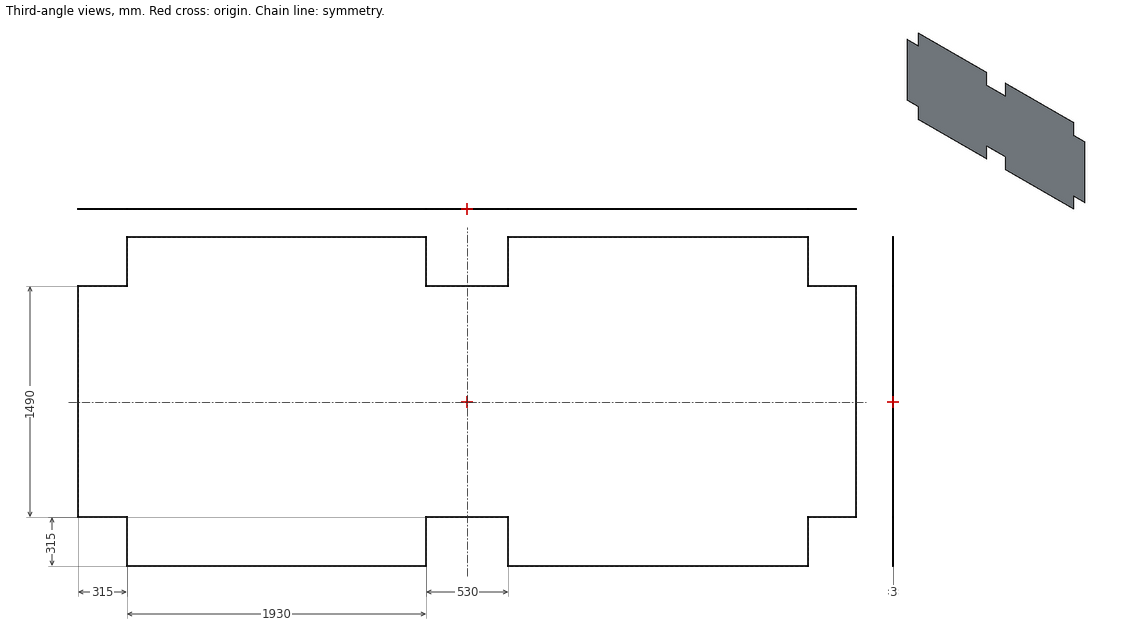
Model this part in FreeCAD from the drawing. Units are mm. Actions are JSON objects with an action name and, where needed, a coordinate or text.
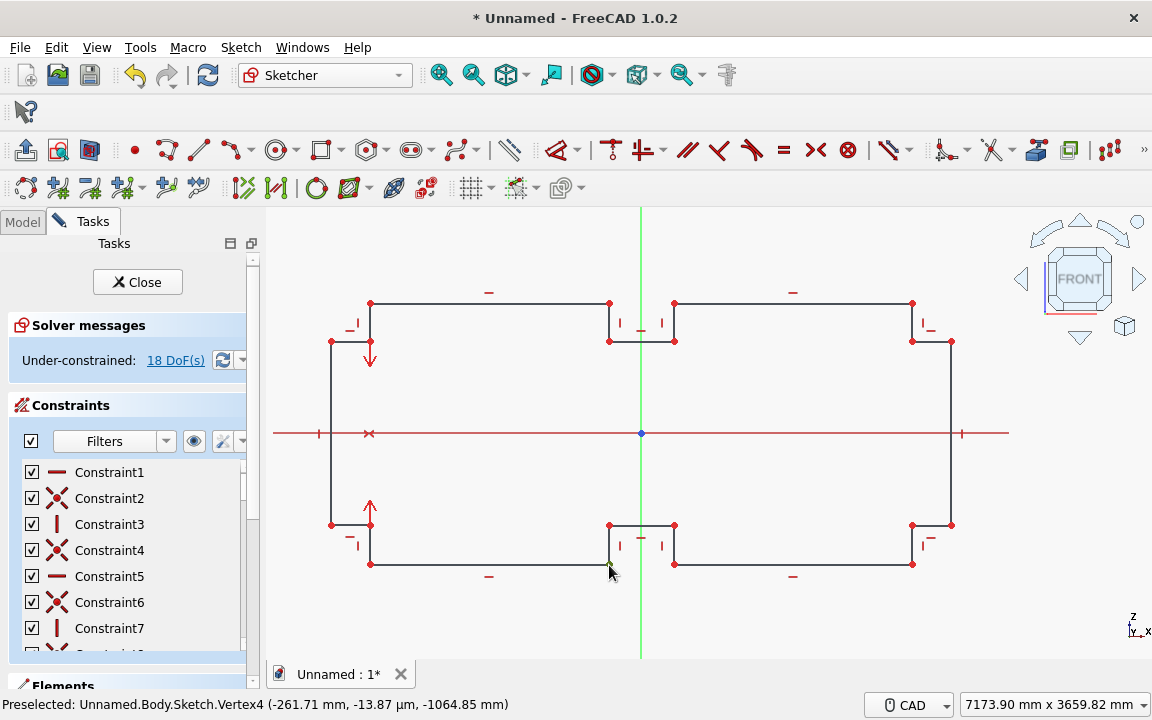
{"action": "left_click", "coordinate": [609, 304]}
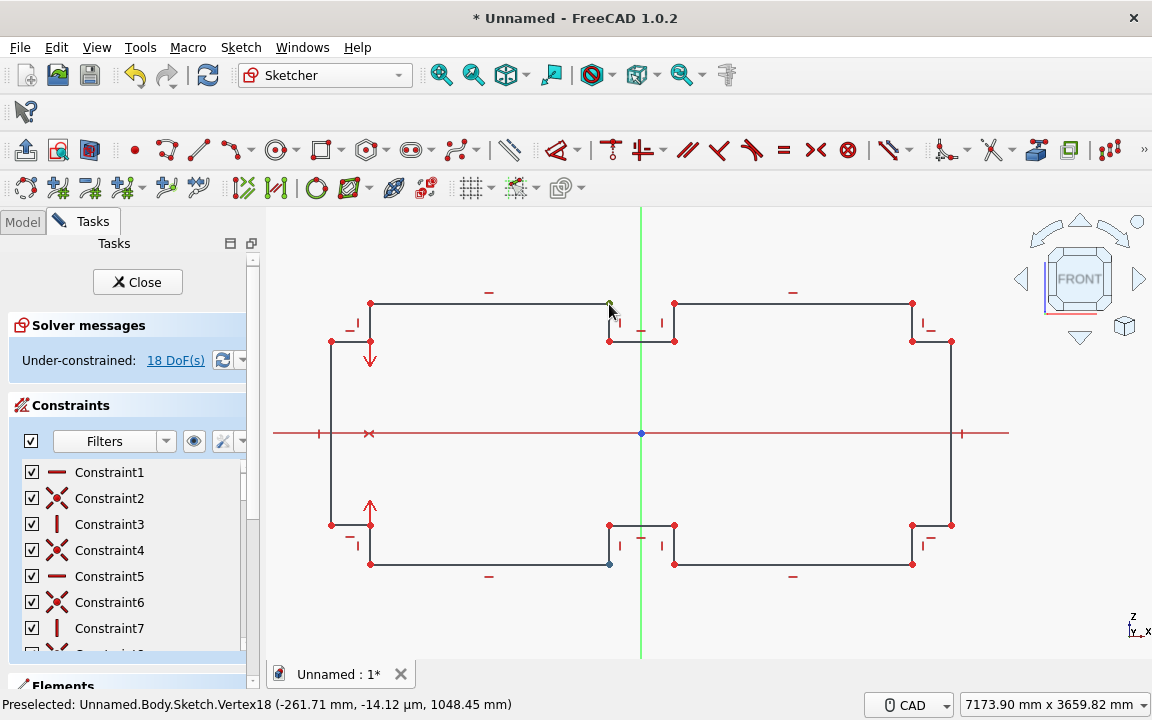
{"action": "left_click", "coordinate": [393, 433]}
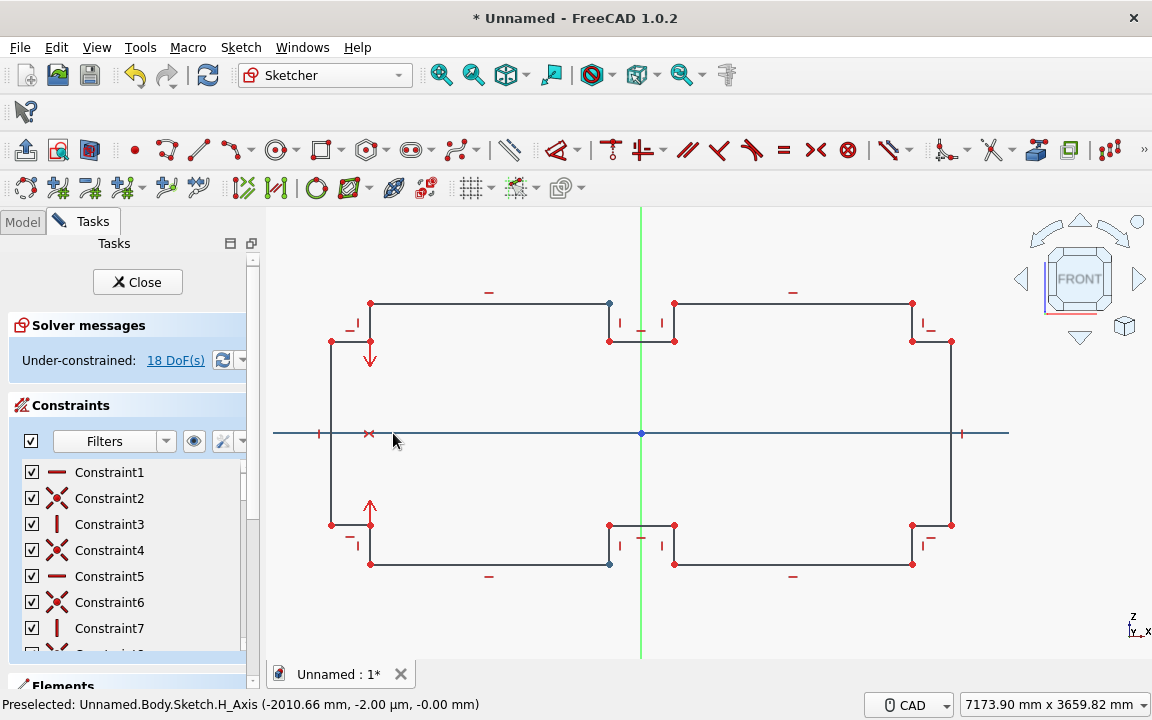
{"action": "left_click", "coordinate": [816, 150]}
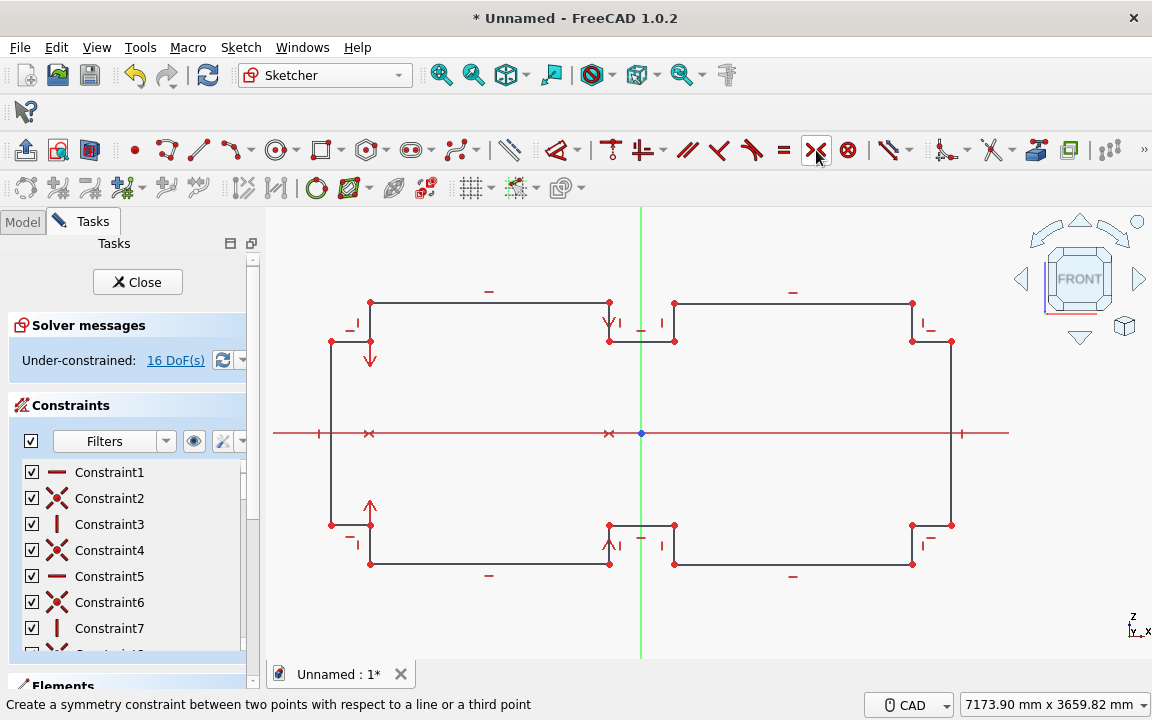
{"action": "left_click", "coordinate": [674, 526]}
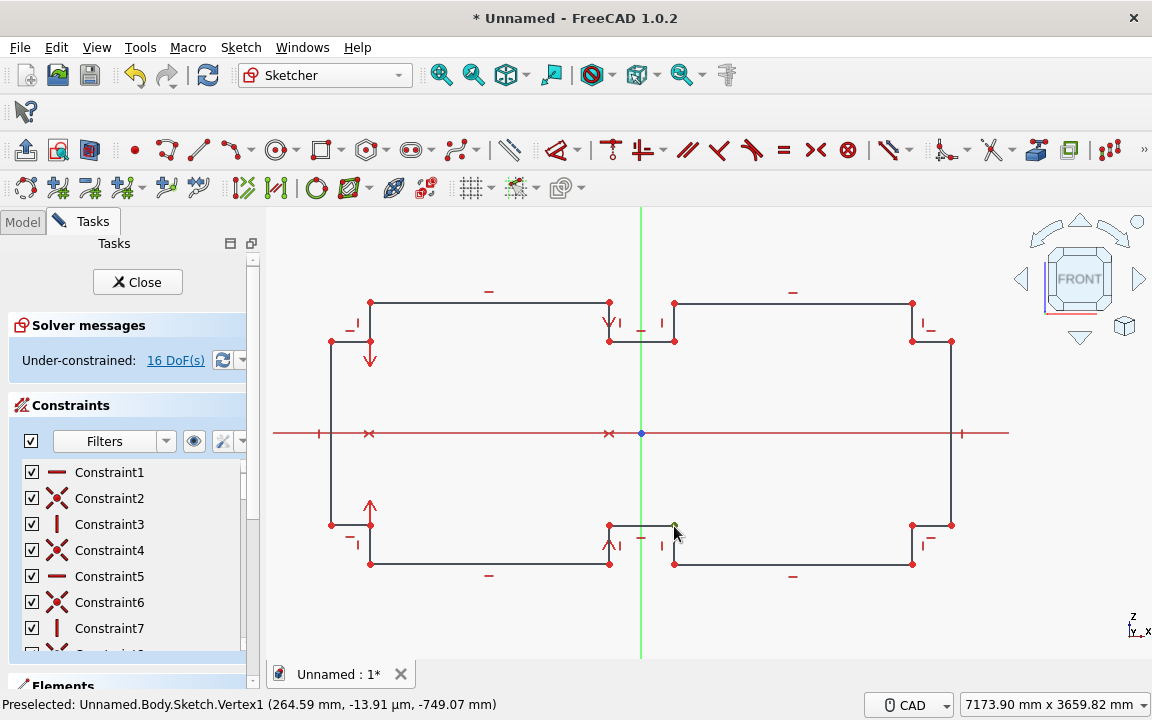
{"action": "left_click", "coordinate": [674, 342]}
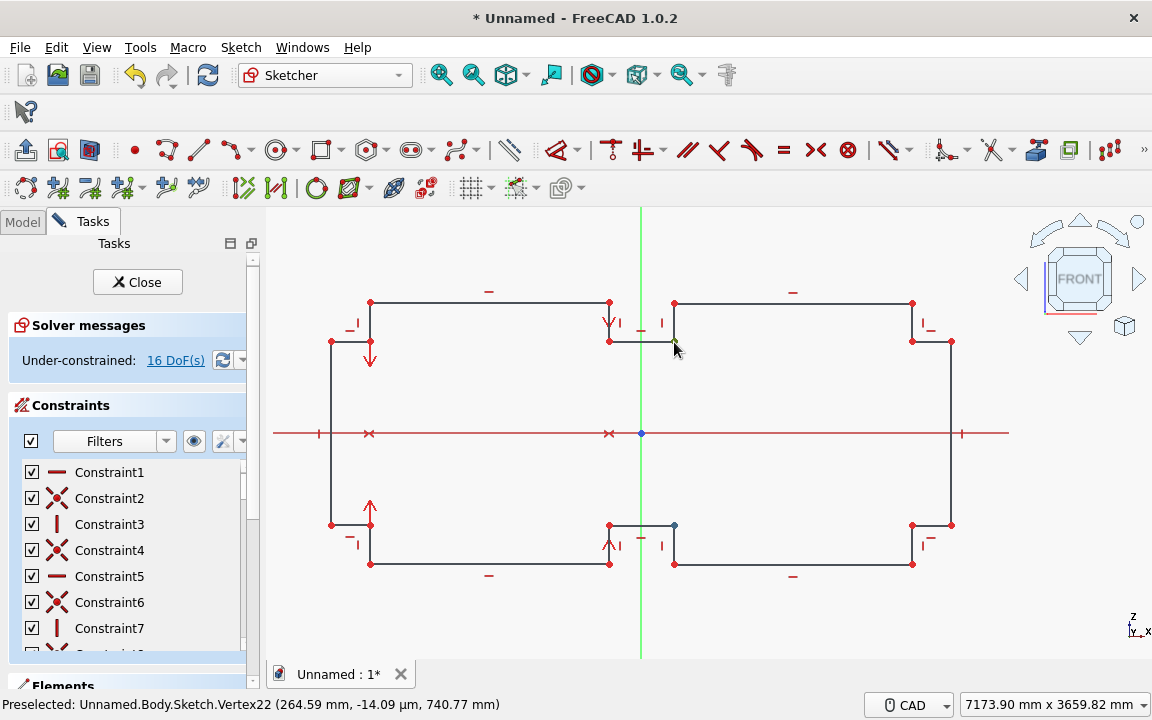
{"action": "left_click", "coordinate": [393, 433]}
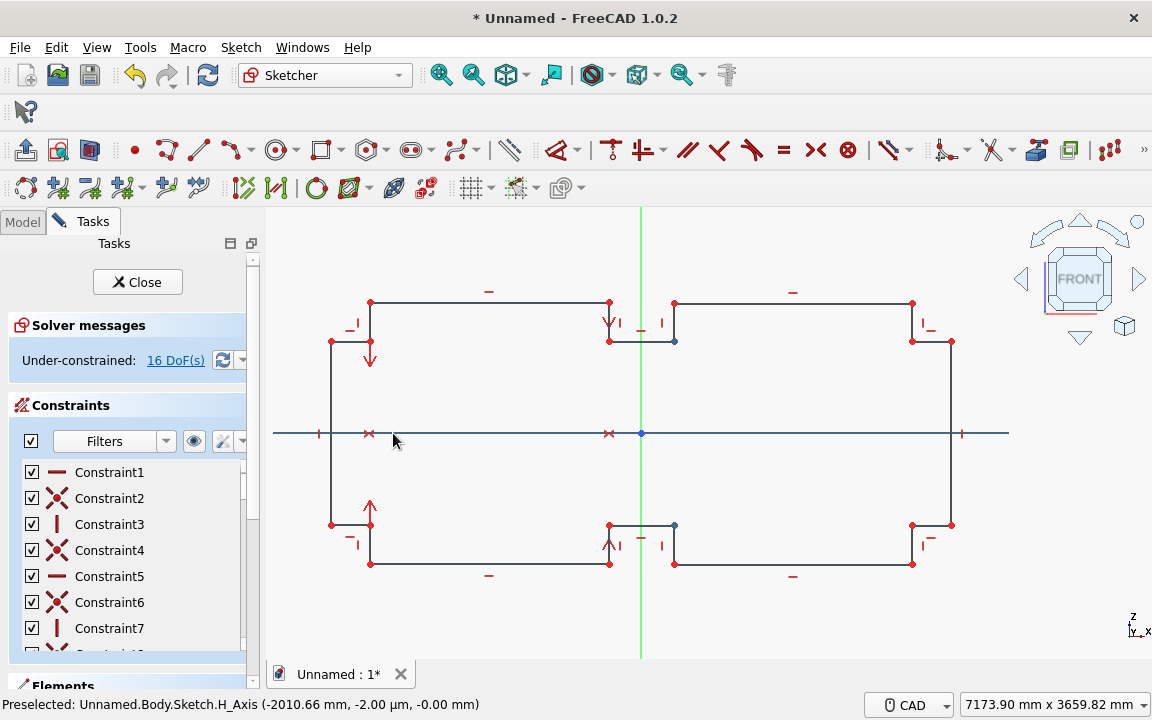
{"action": "left_click", "coordinate": [816, 150]}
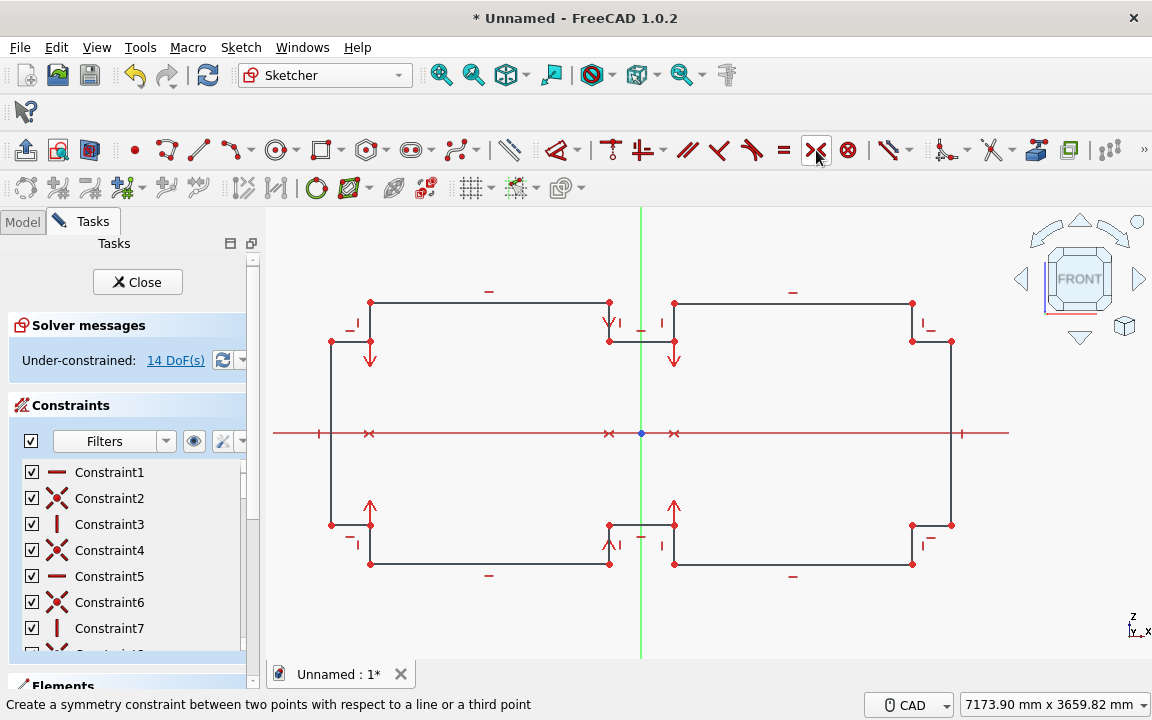
{"action": "left_click", "coordinate": [609, 303]}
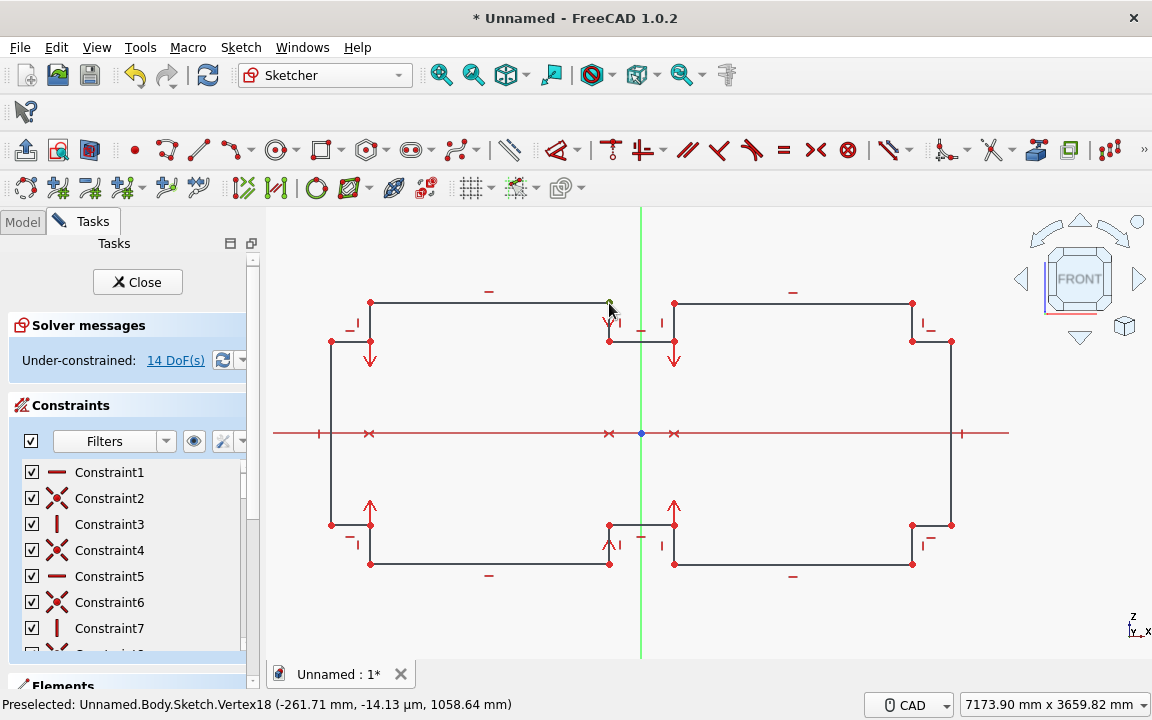
{"action": "left_click", "coordinate": [674, 304]}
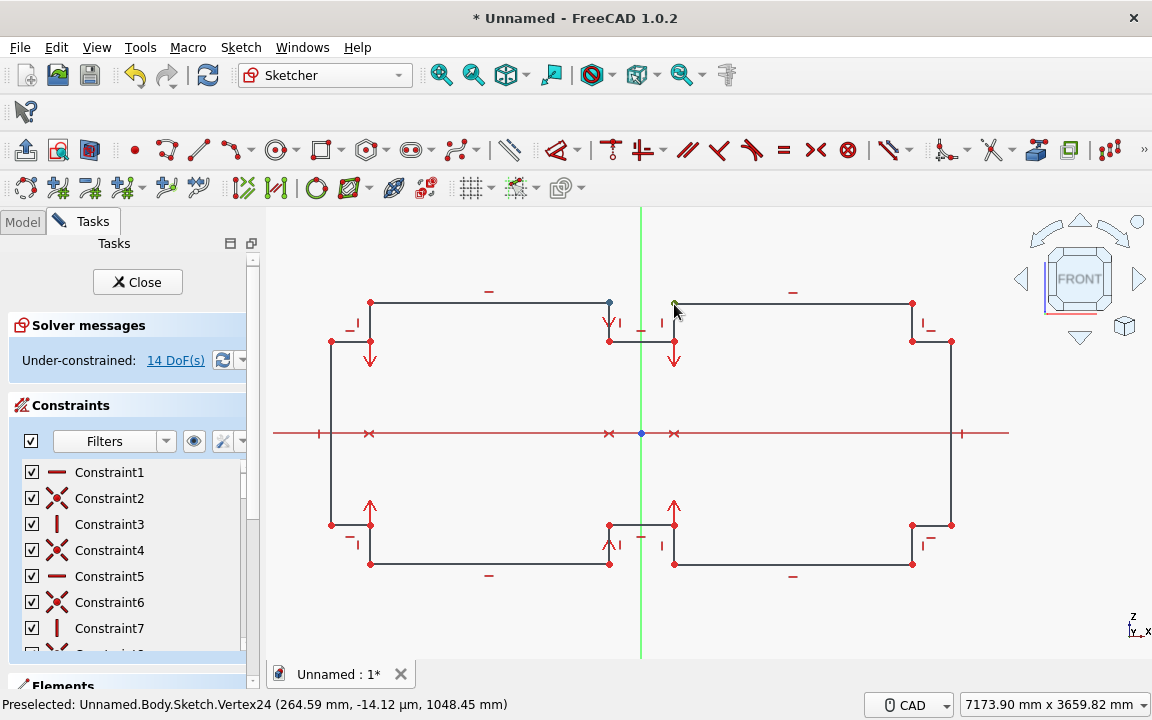
{"action": "left_click", "coordinate": [641, 603]}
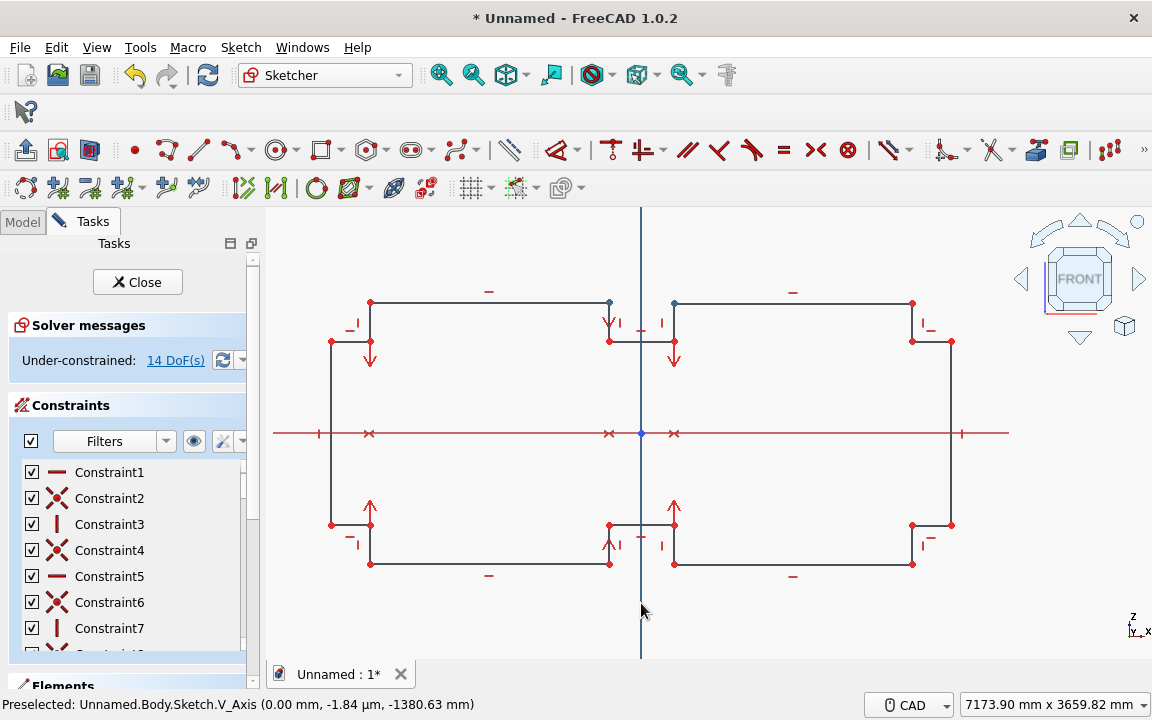
{"action": "left_click", "coordinate": [816, 150]}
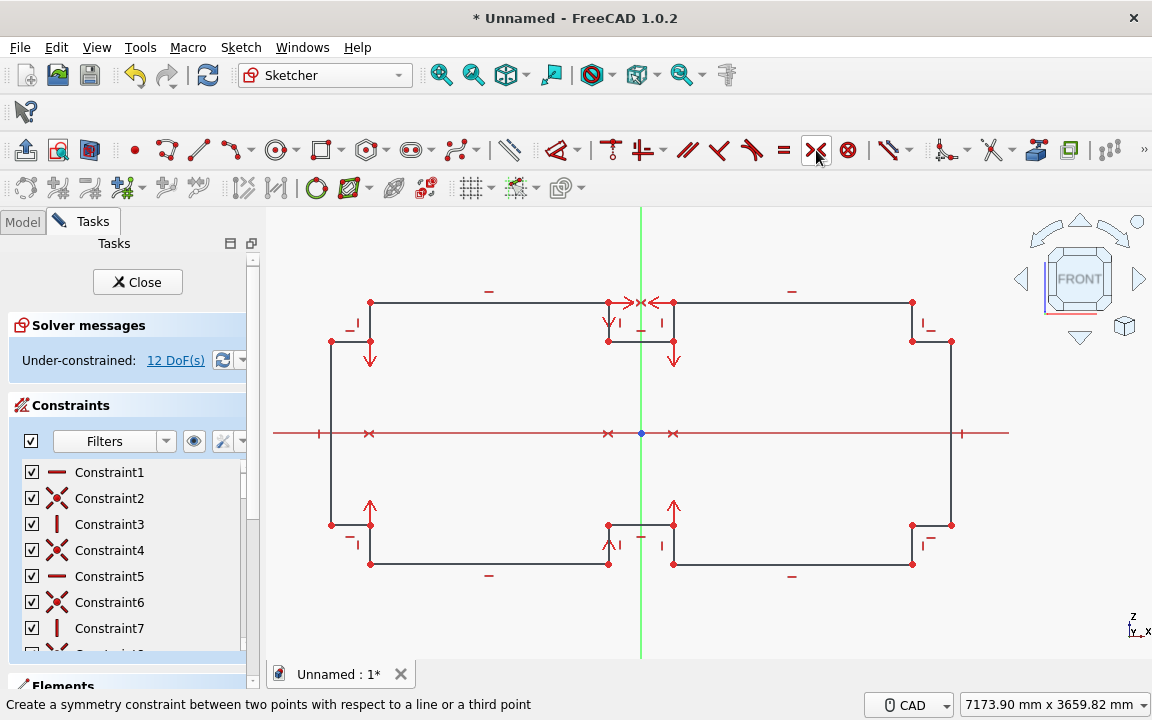
{"action": "left_click", "coordinate": [370, 342]}